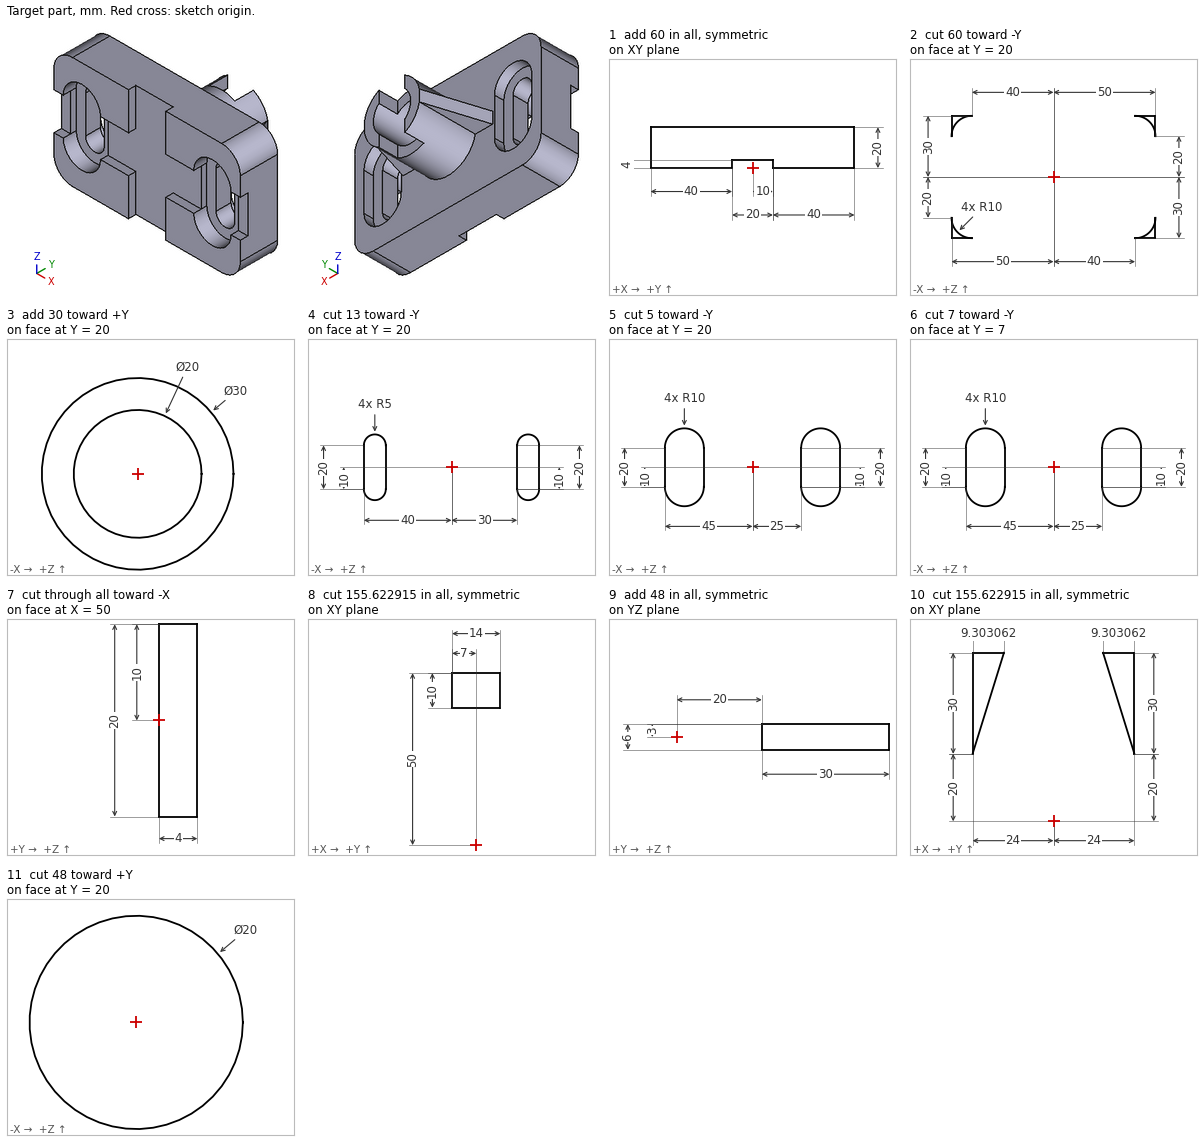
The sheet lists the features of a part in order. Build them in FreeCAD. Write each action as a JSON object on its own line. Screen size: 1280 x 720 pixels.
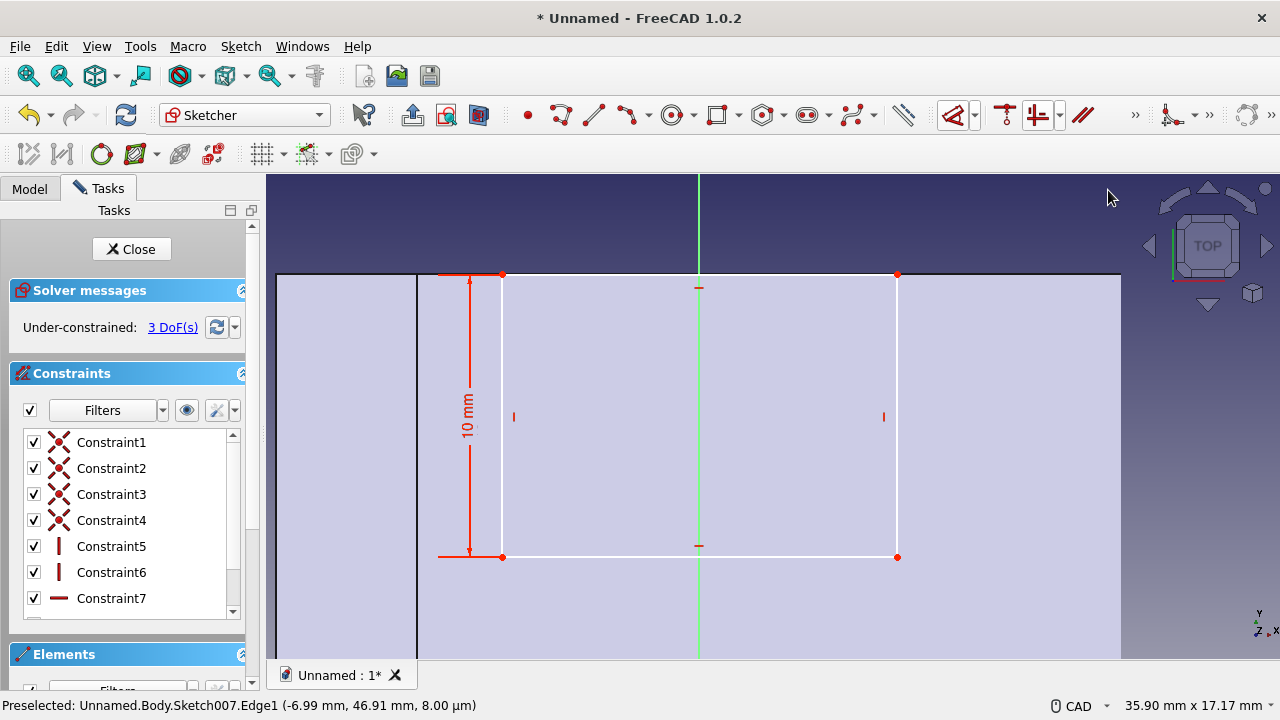
{"action": "left_click", "coordinate": [621, 557]}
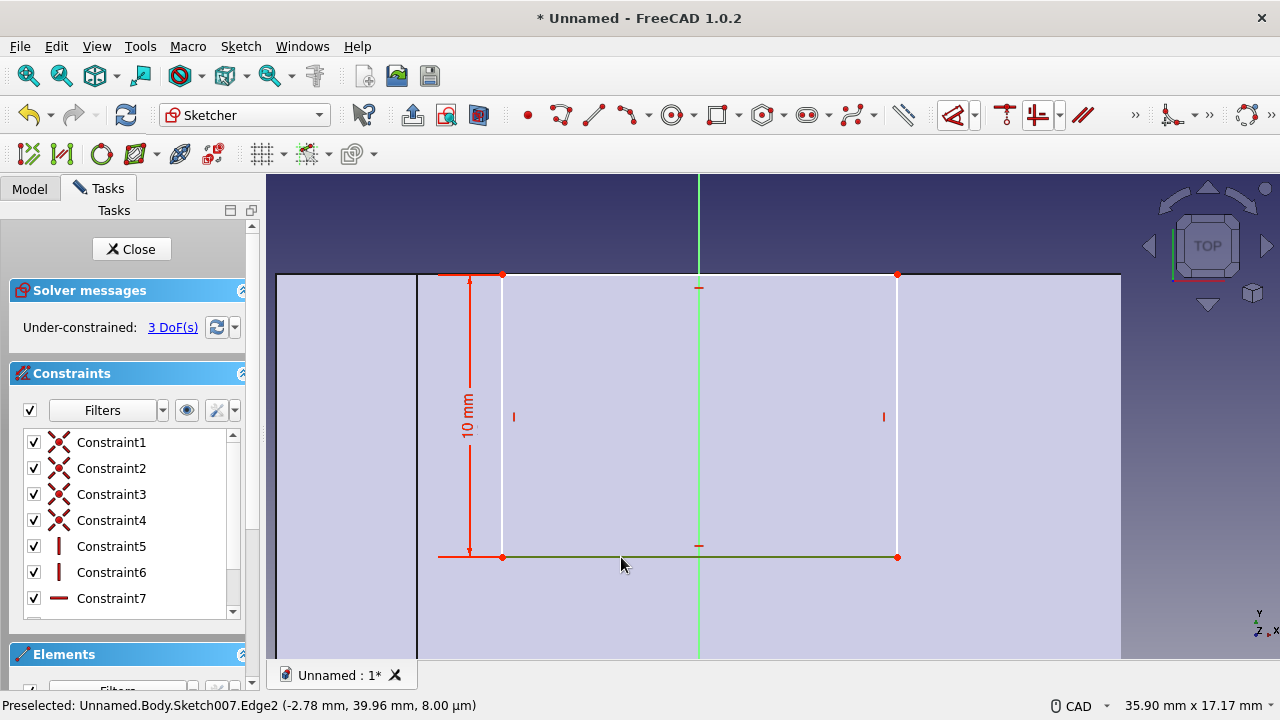
{"action": "key", "text": "l"}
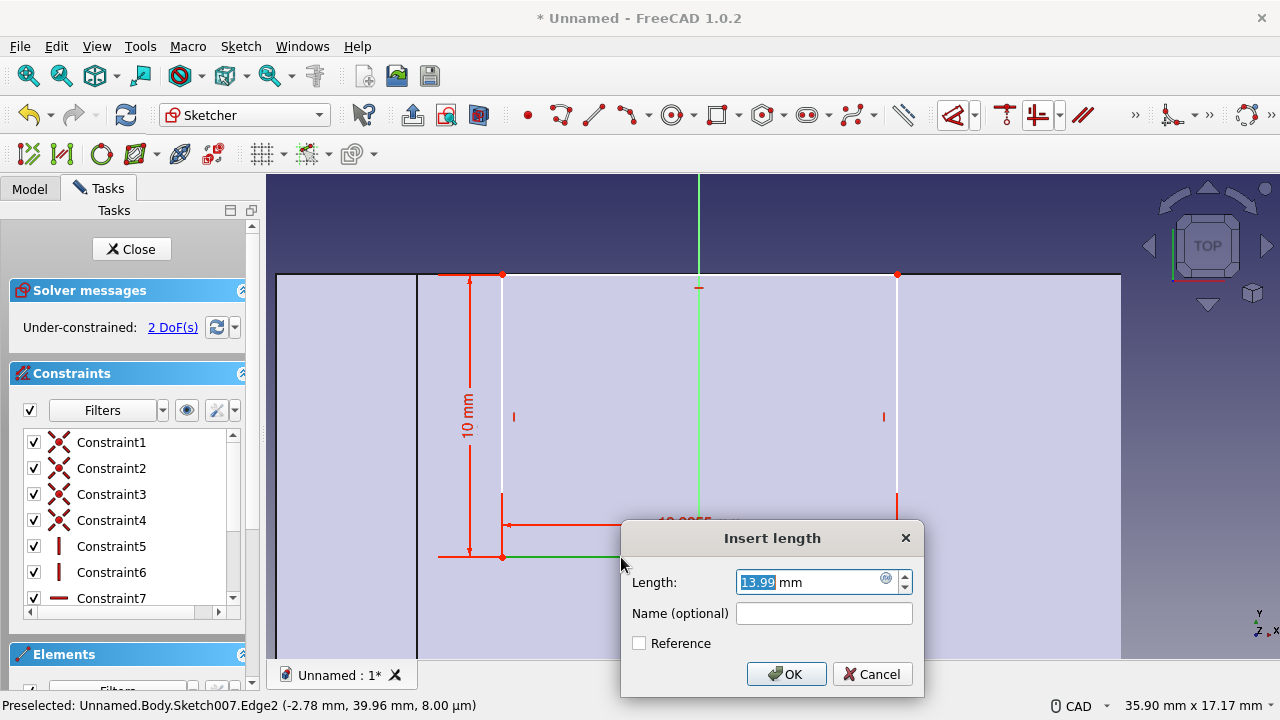
{"action": "type", "text": "14"}
{"action": "key", "text": "Return"}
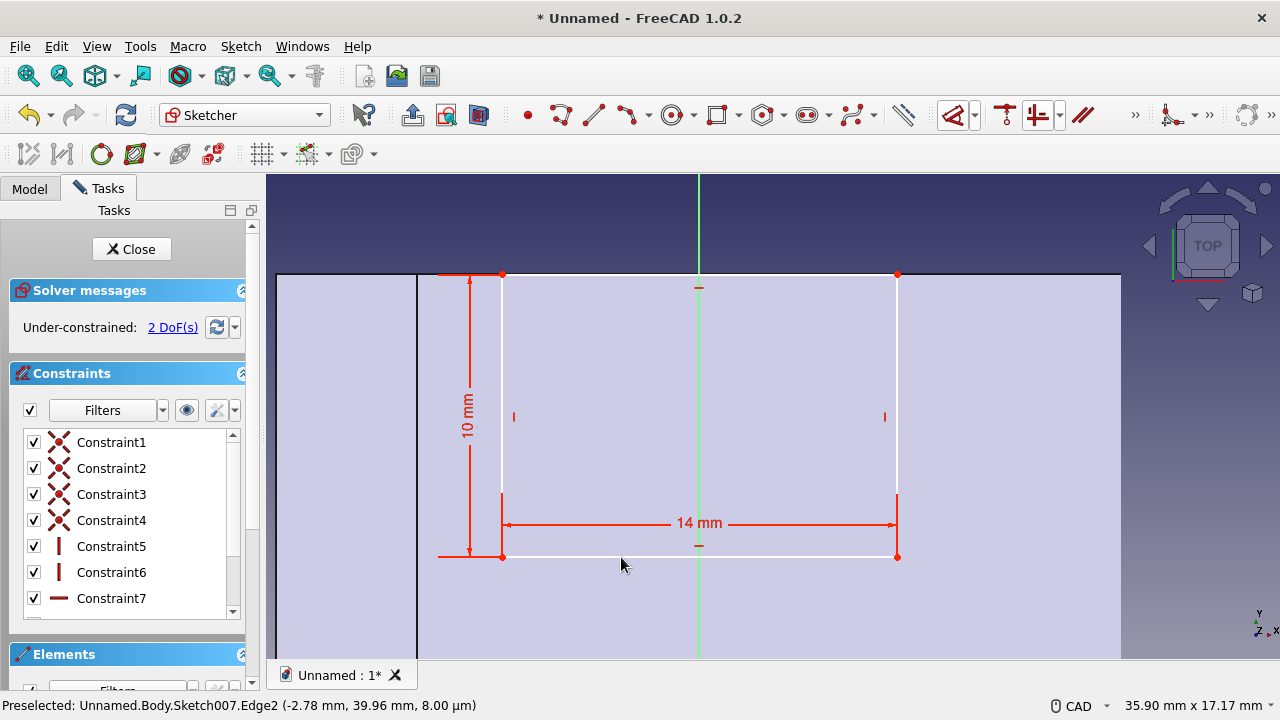
{"action": "left_click", "coordinate": [502, 275]}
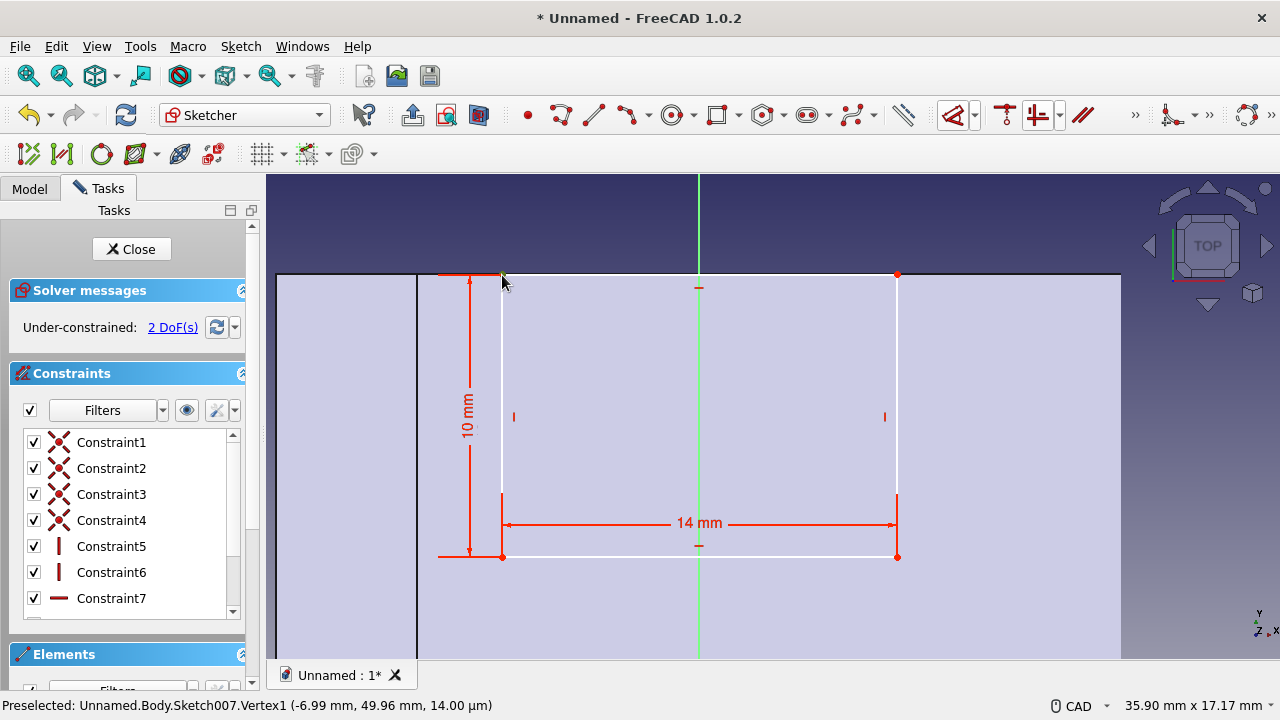
{"action": "key", "text": "l"}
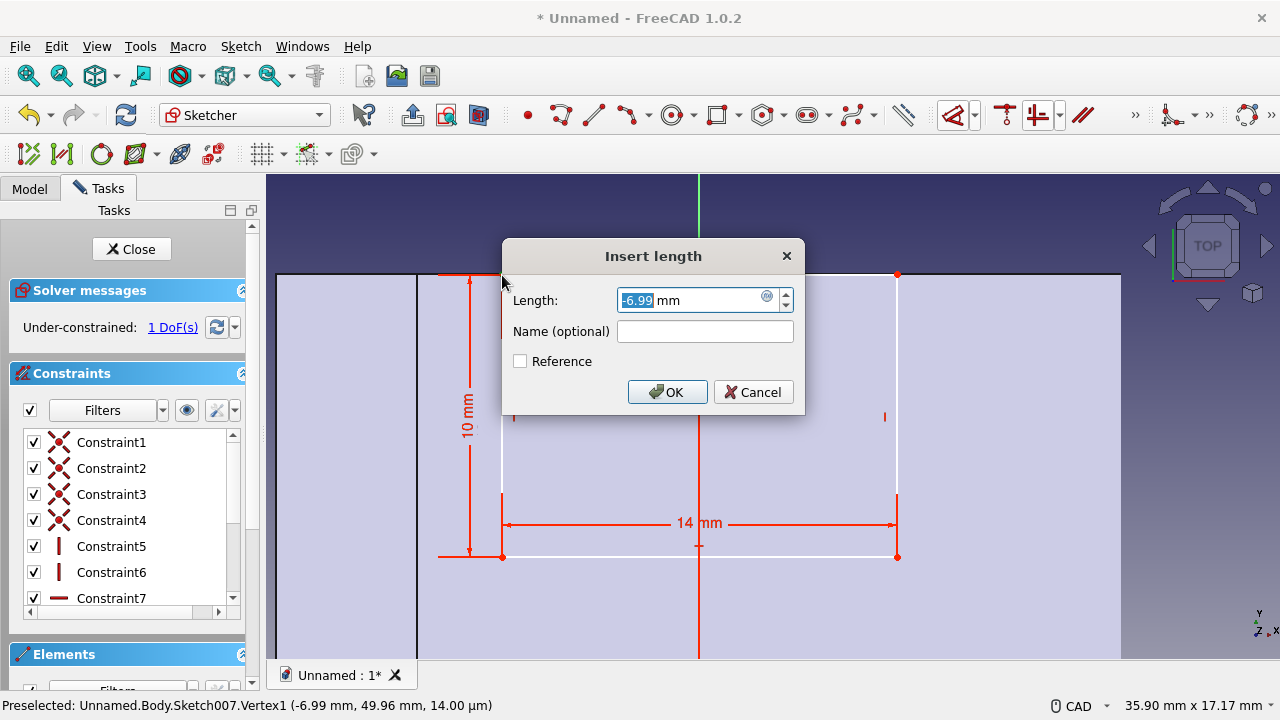
{"action": "type", "text": "-7"}
{"action": "key", "text": "Return"}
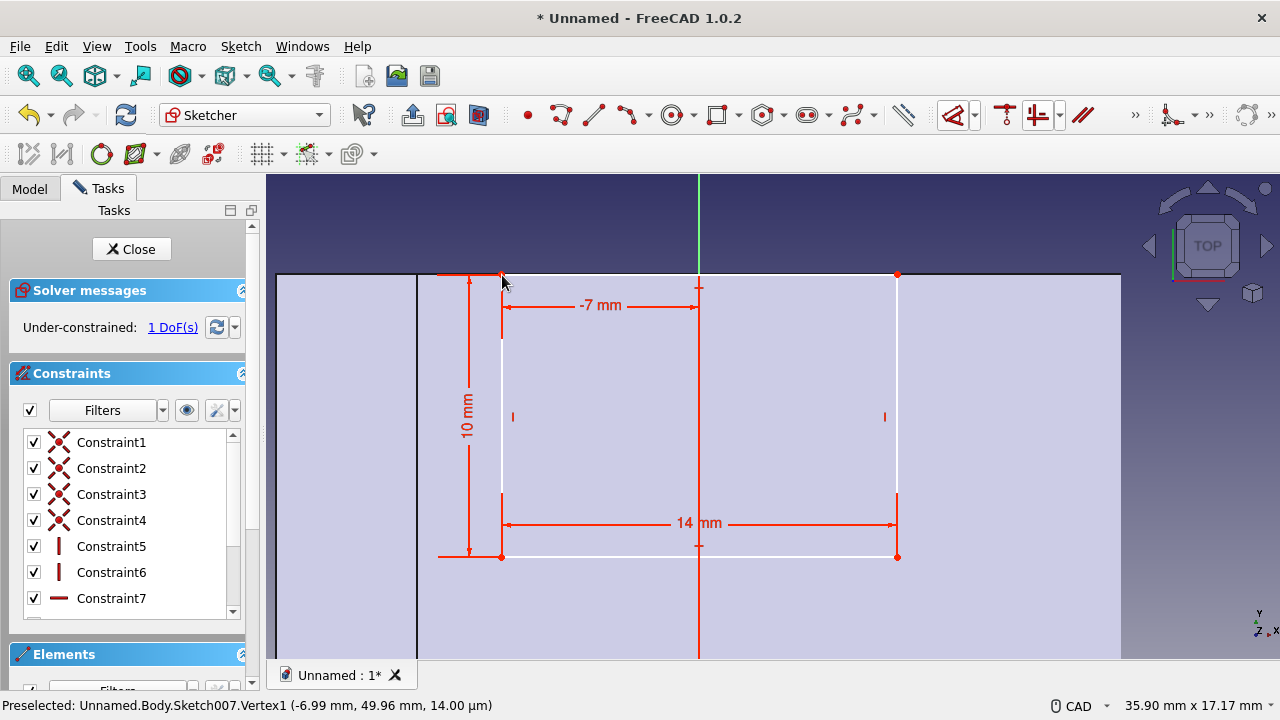
{"action": "left_click", "coordinate": [502, 275]}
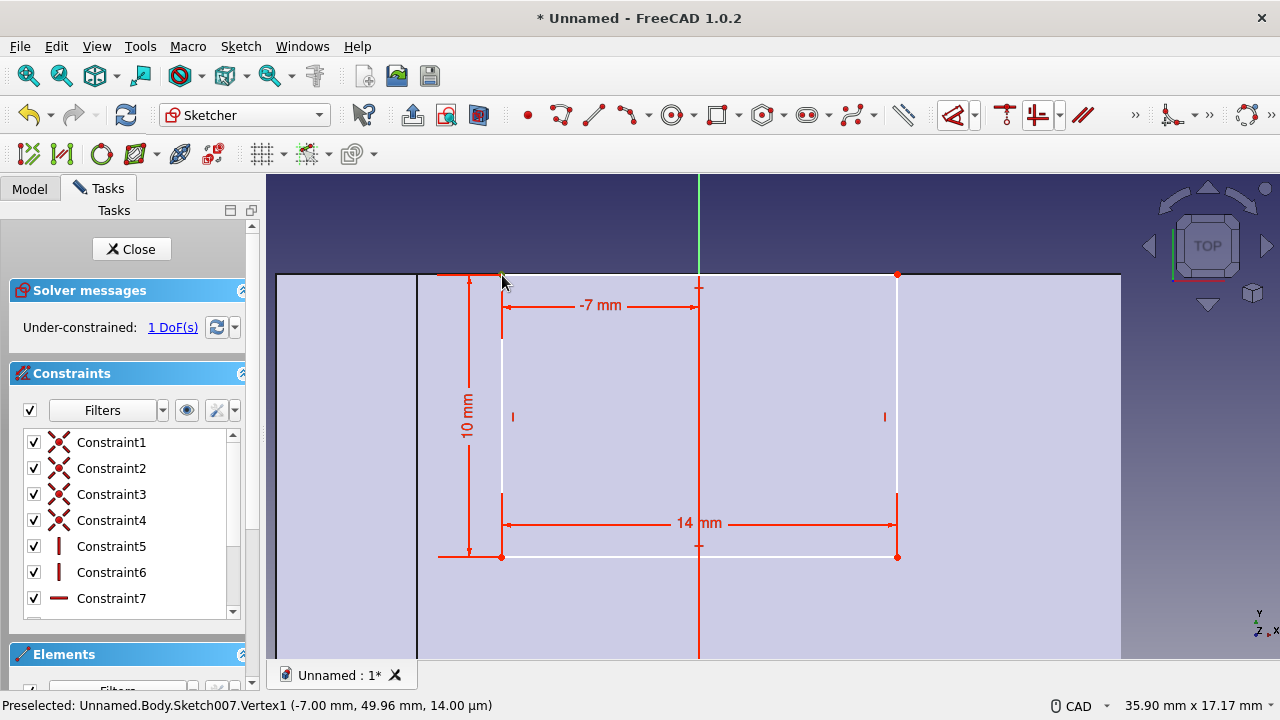
{"action": "key", "text": "i"}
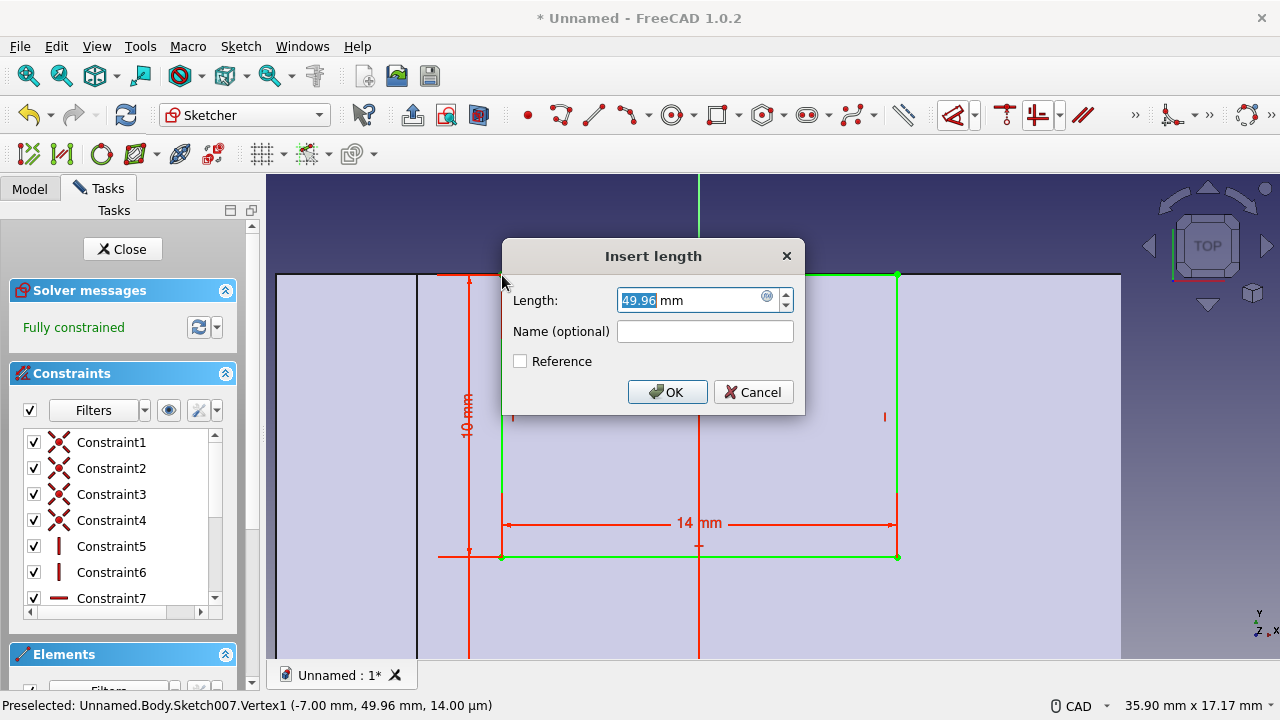
{"action": "type", "text": "50"}
{"action": "key", "text": "Return"}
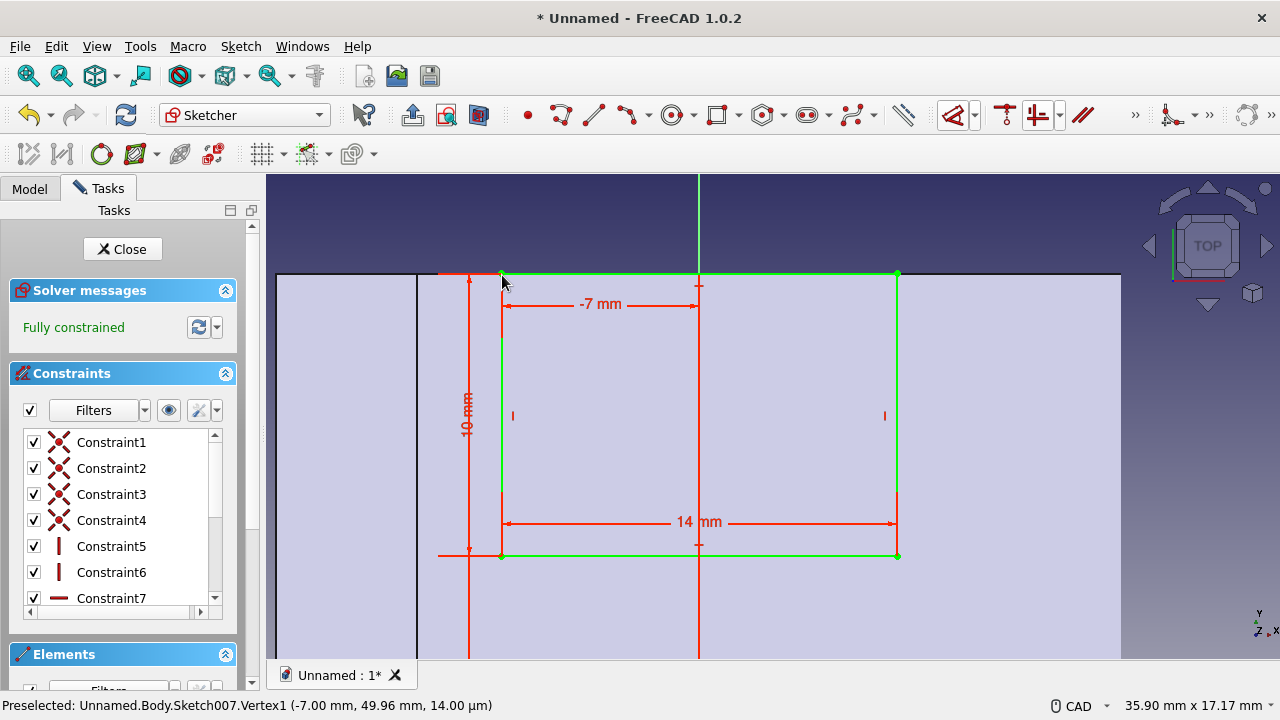
{"action": "left_click", "coordinate": [123, 249]}